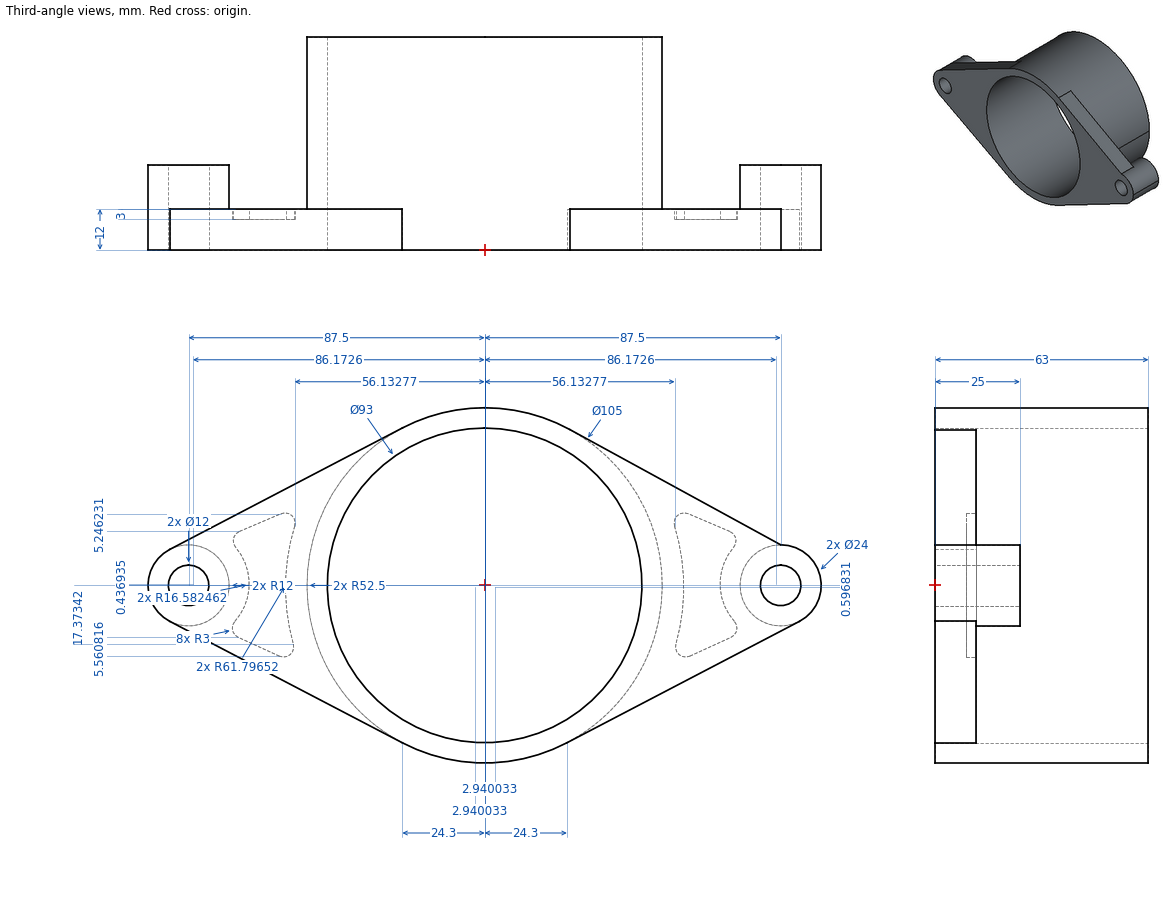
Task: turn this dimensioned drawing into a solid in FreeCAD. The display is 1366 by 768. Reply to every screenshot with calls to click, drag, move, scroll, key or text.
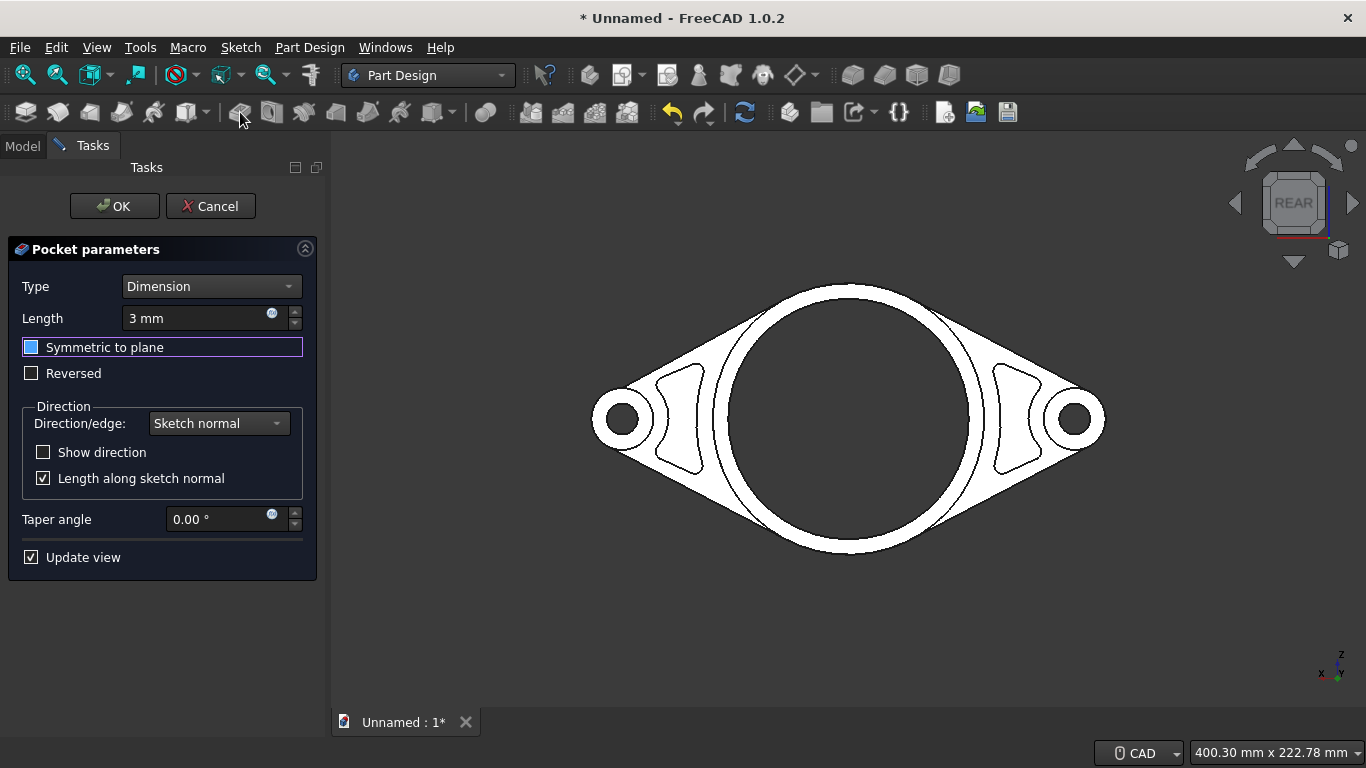
click(115, 206)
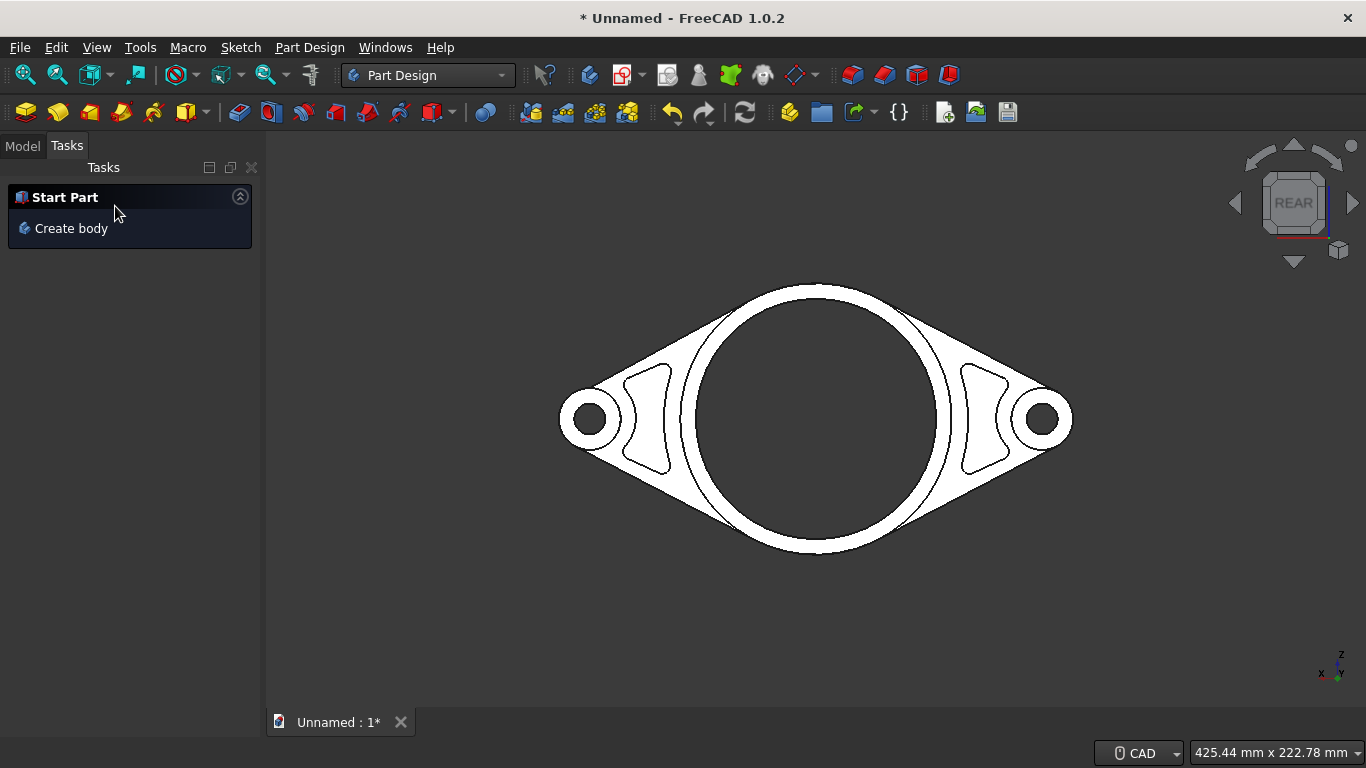
key(0)